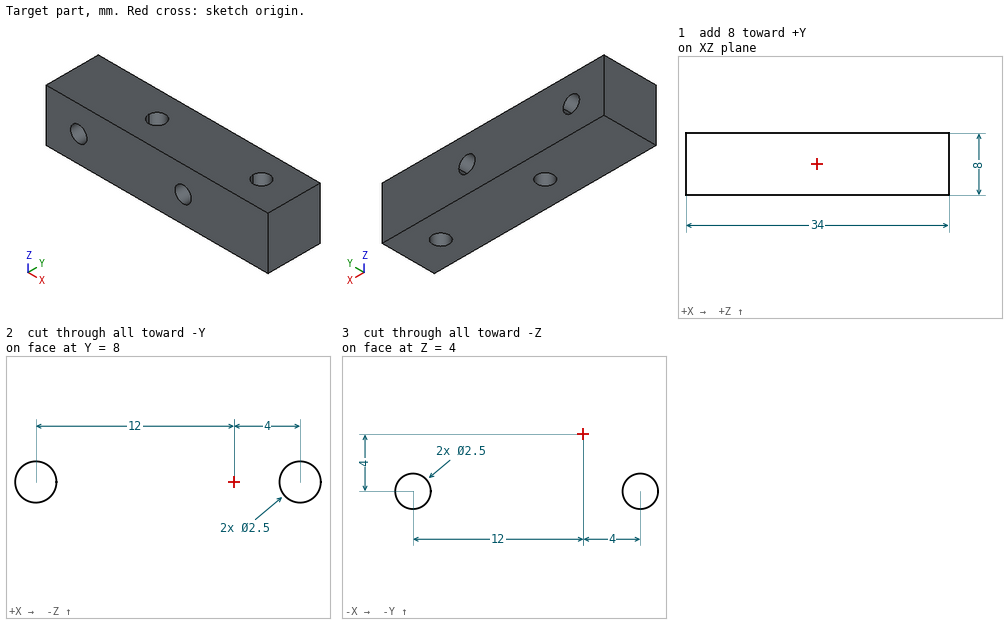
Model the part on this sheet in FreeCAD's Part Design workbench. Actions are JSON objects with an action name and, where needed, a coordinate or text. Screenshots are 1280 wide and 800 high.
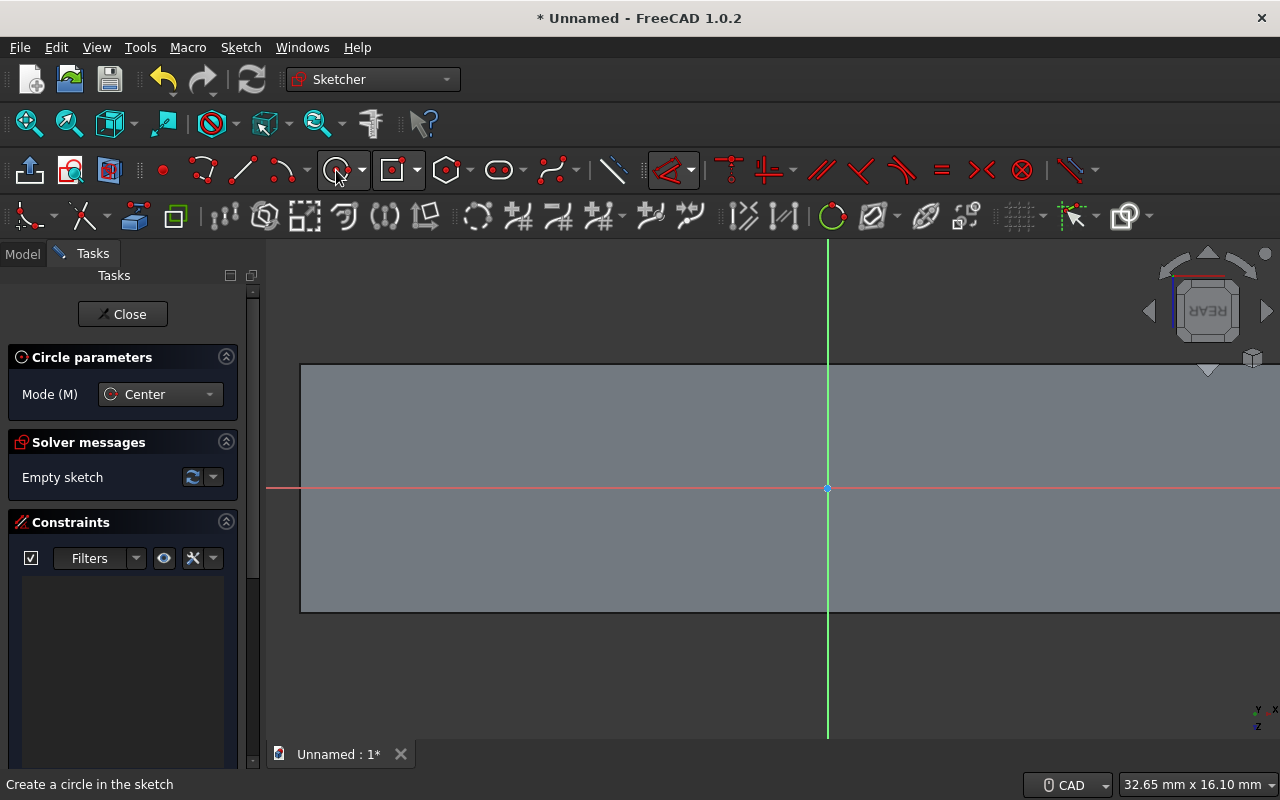
{"action": "left_click", "coordinate": [952, 488]}
{"action": "mouse_move", "coordinate": [979, 461]}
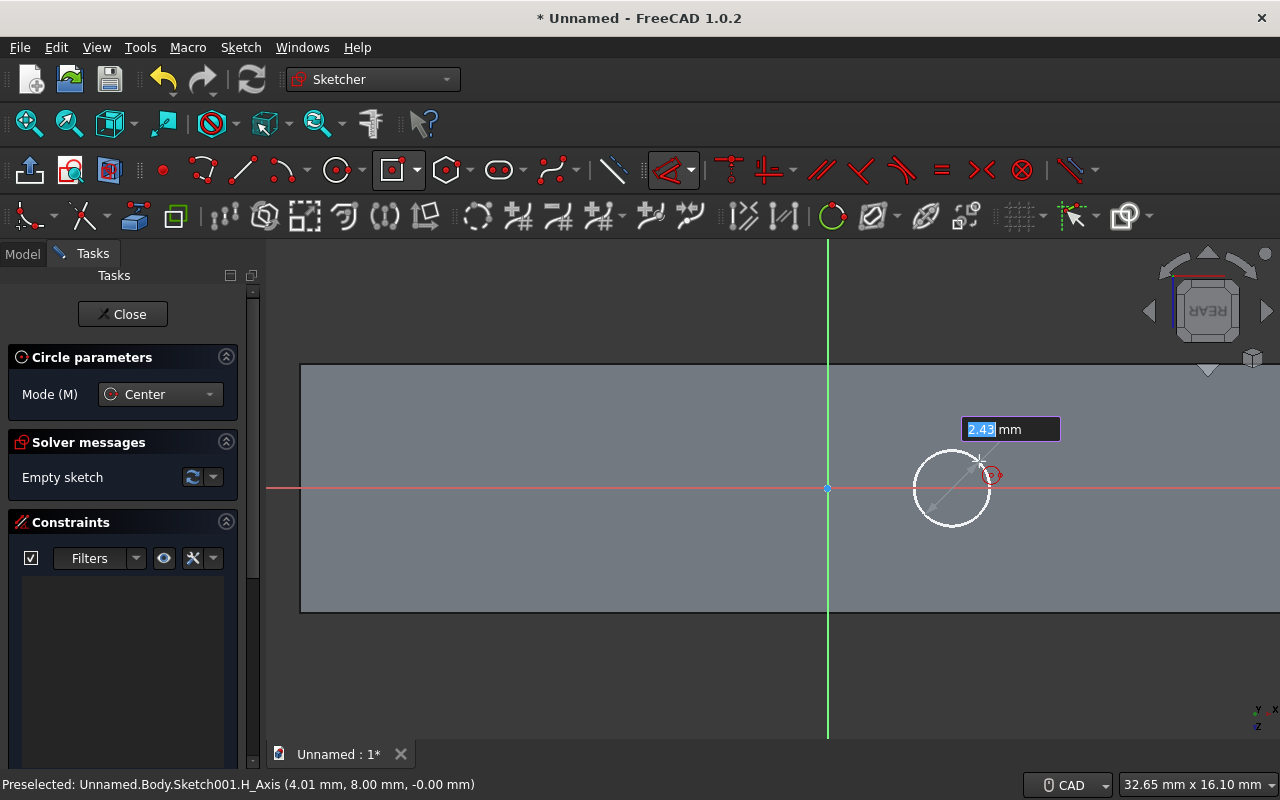
{"action": "type", "text": "2.5"}
{"action": "key", "text": "Return"}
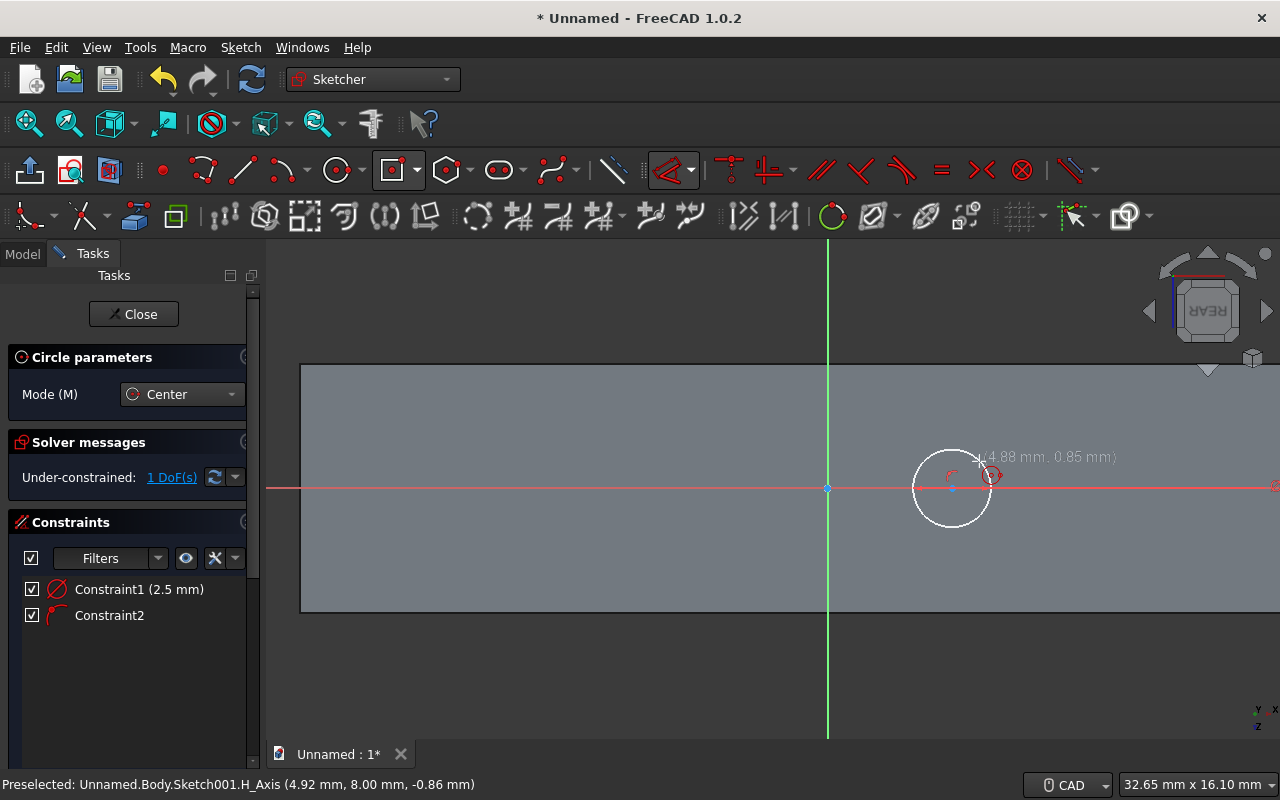
{"action": "left_click", "coordinate": [455, 488]}
{"action": "mouse_move", "coordinate": [482, 461]}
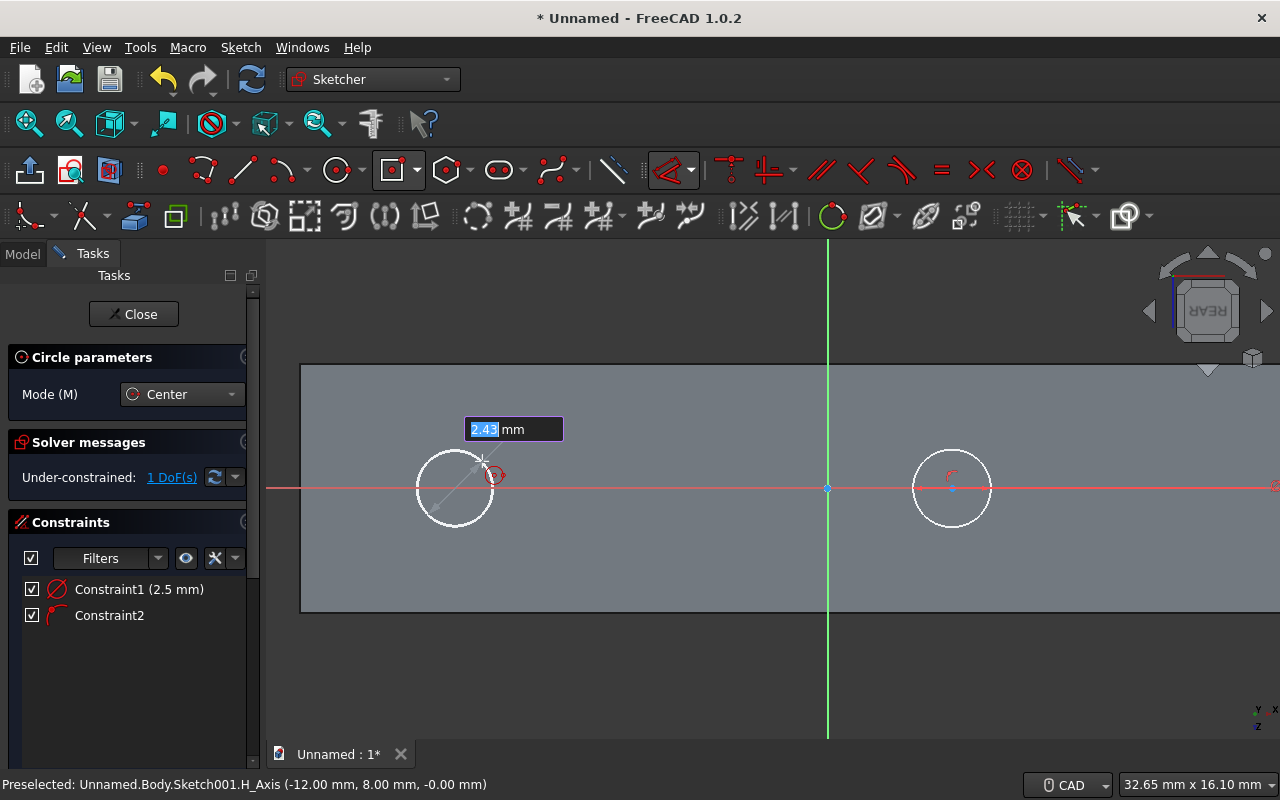
{"action": "type", "text": "2.5"}
{"action": "key", "text": "Return"}
{"action": "key", "text": "Escape"}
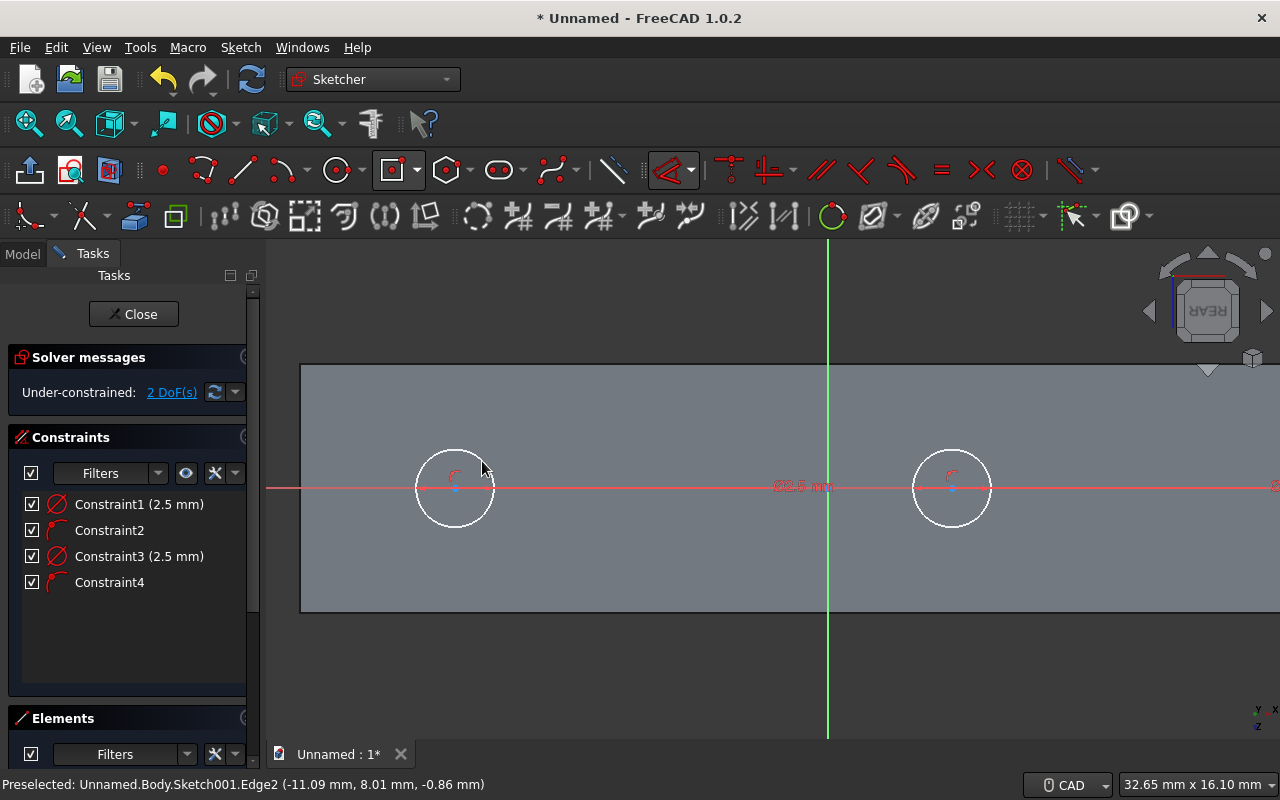
{"action": "left_click", "coordinate": [668, 170]}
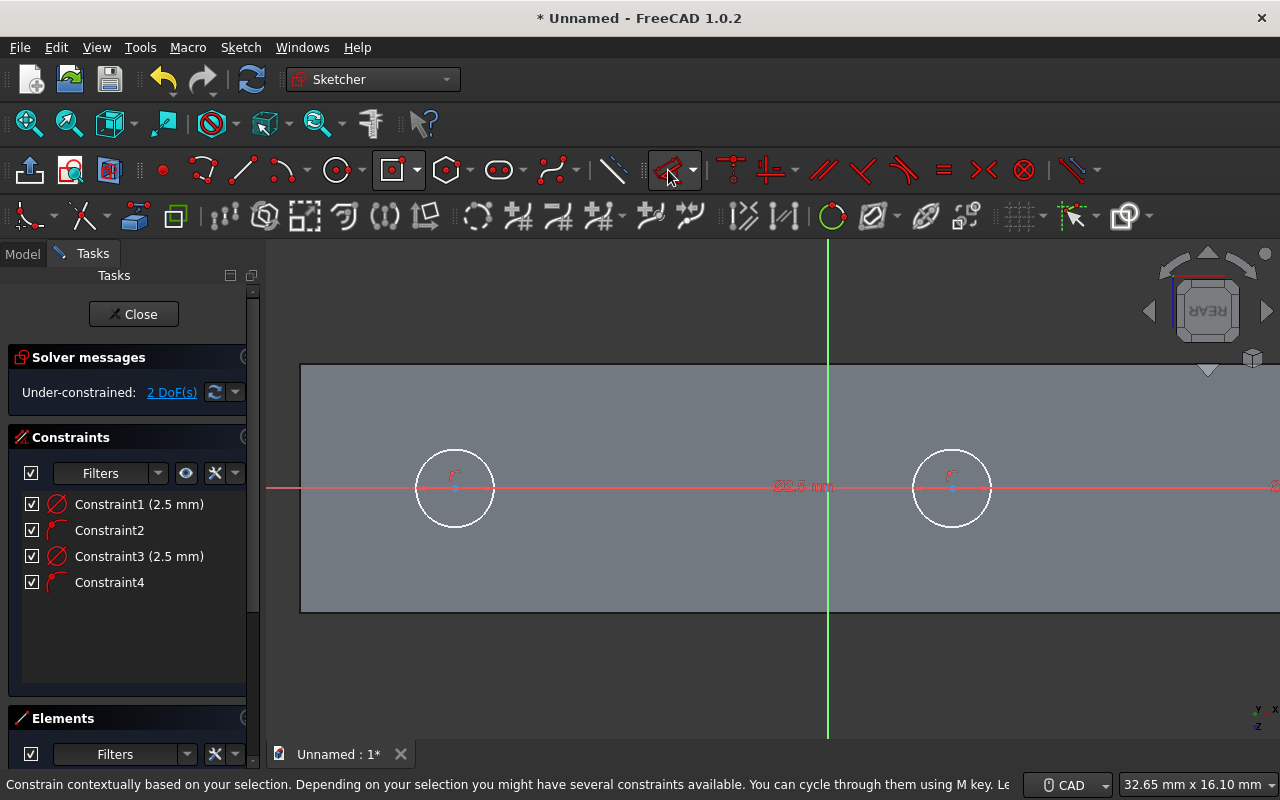
{"action": "left_click", "coordinate": [952, 488]}
{"action": "left_click", "coordinate": [890, 522]}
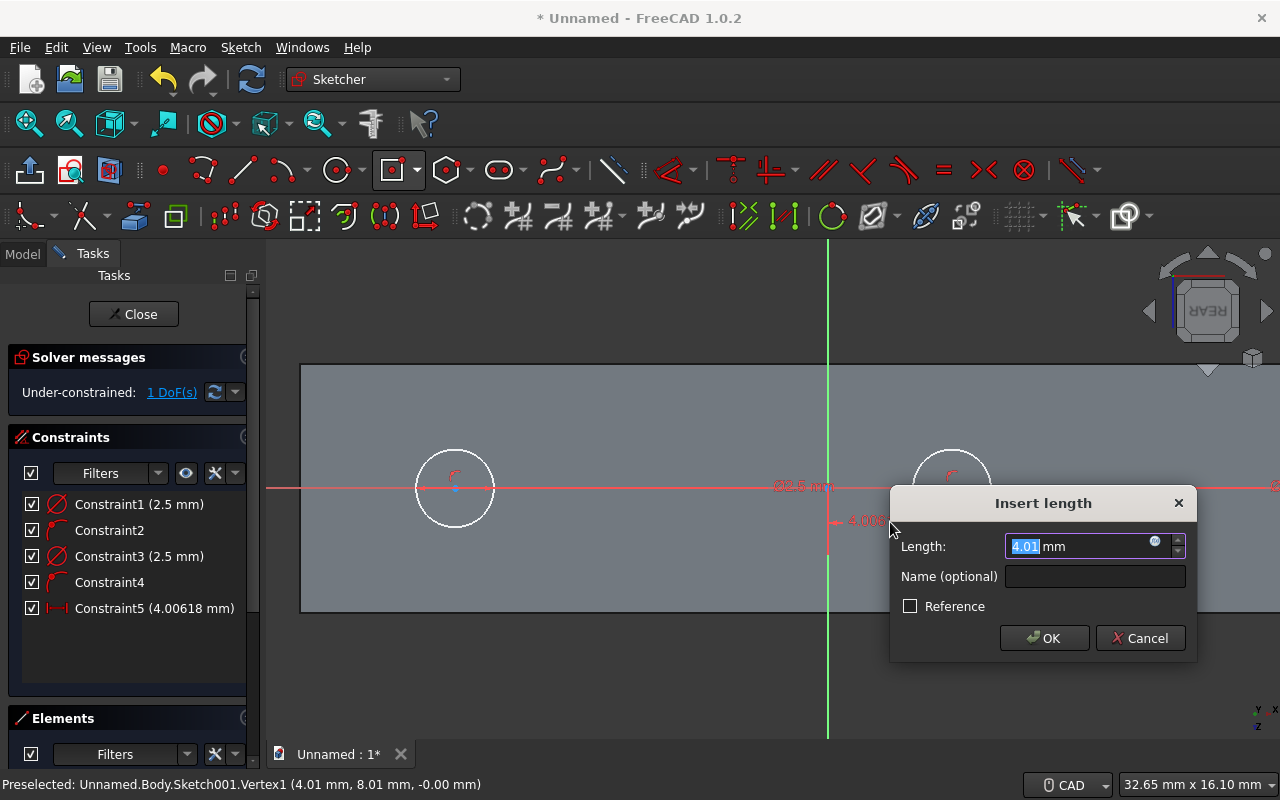
{"action": "type", "text": "4"}
{"action": "key", "text": "Return"}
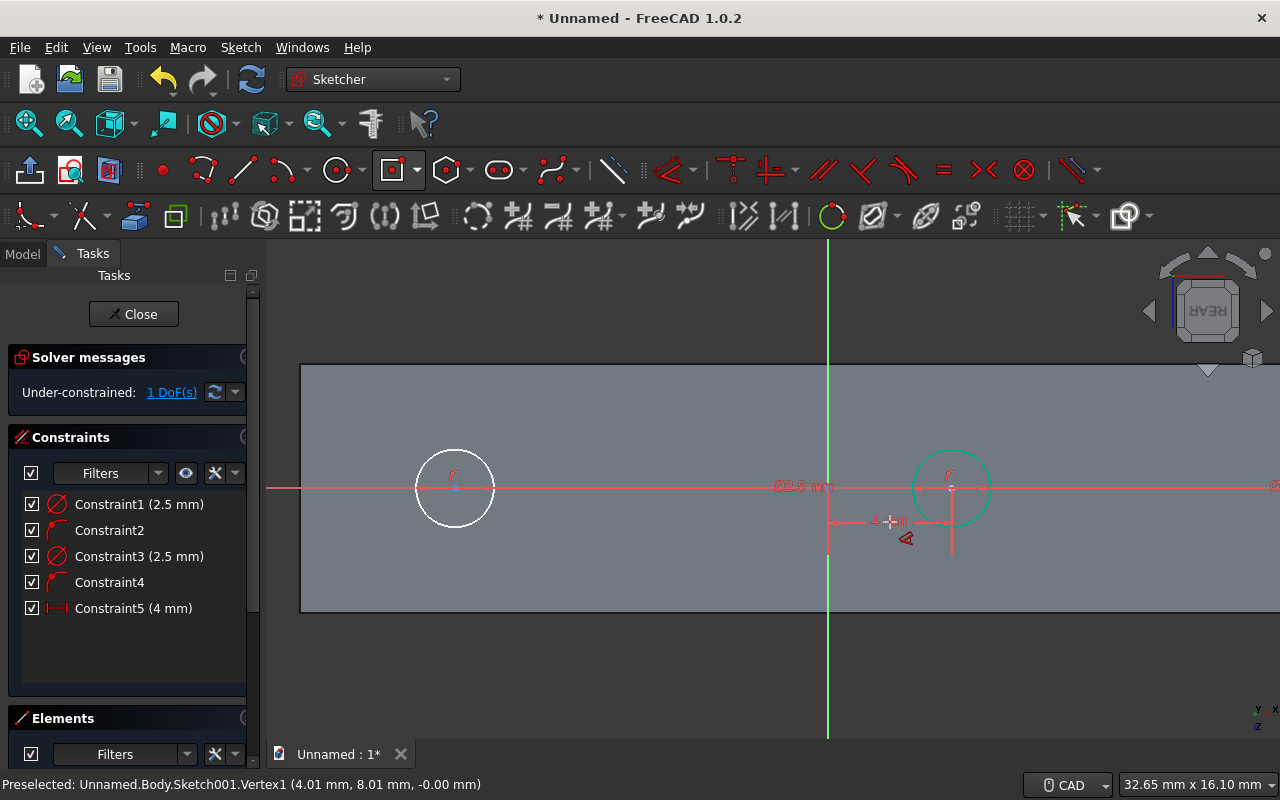
{"action": "left_click", "coordinate": [455, 488]}
{"action": "left_click", "coordinate": [641, 522]}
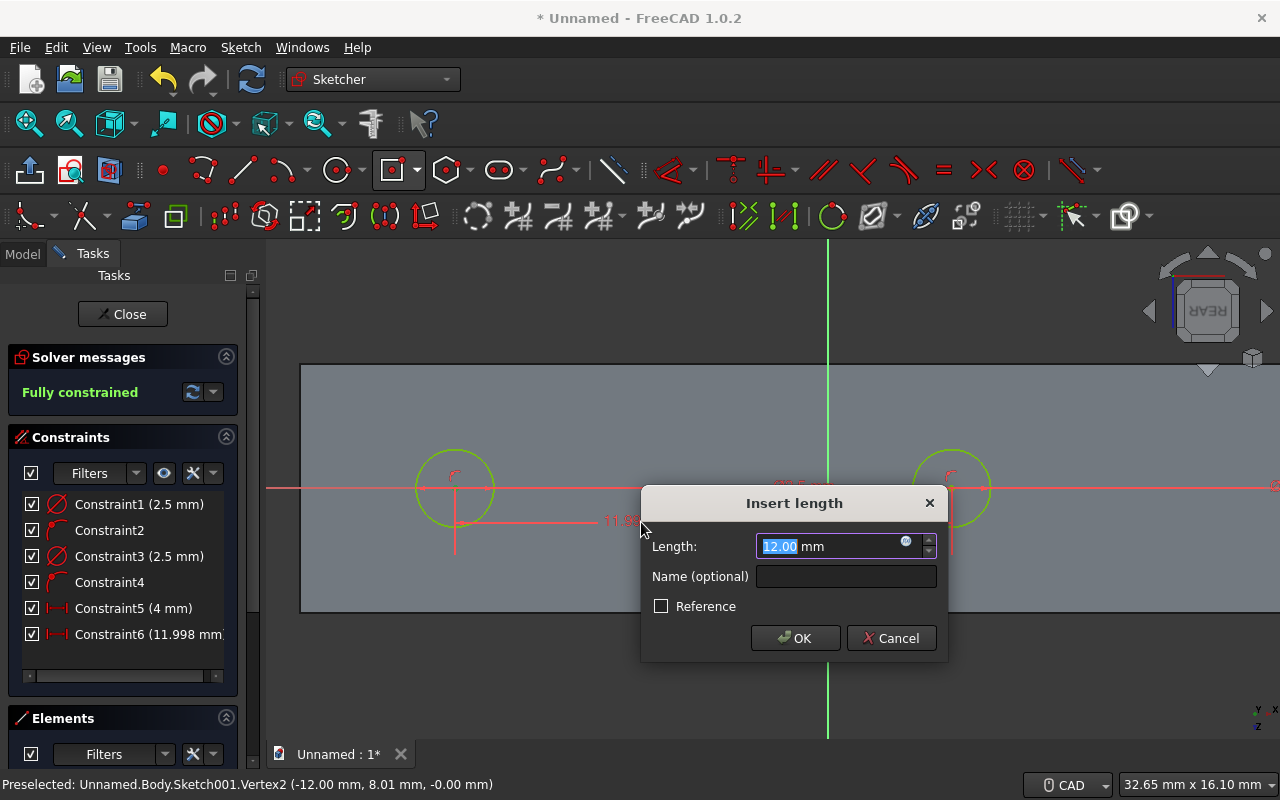
{"action": "type", "text": "12"}
{"action": "key", "text": "Return"}
{"action": "key", "text": "Escape"}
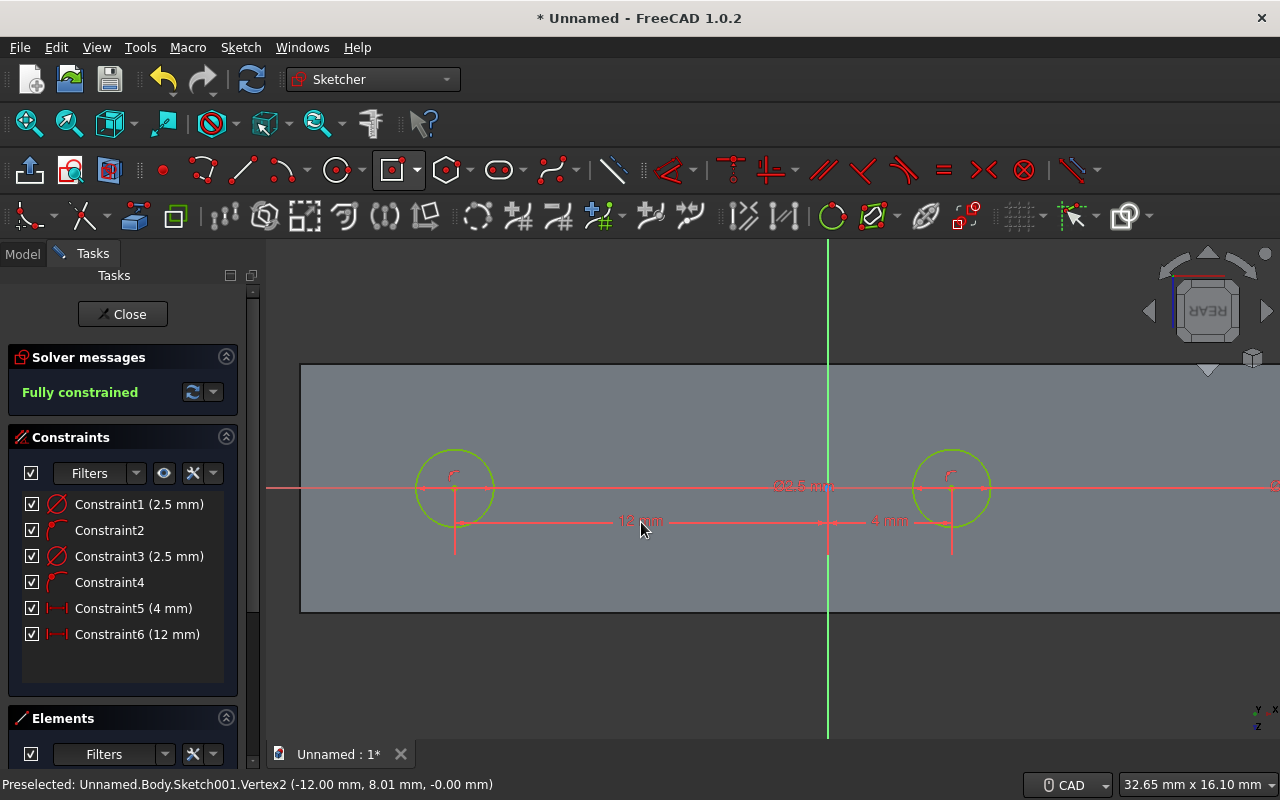
{"action": "left_click", "coordinate": [123, 314]}